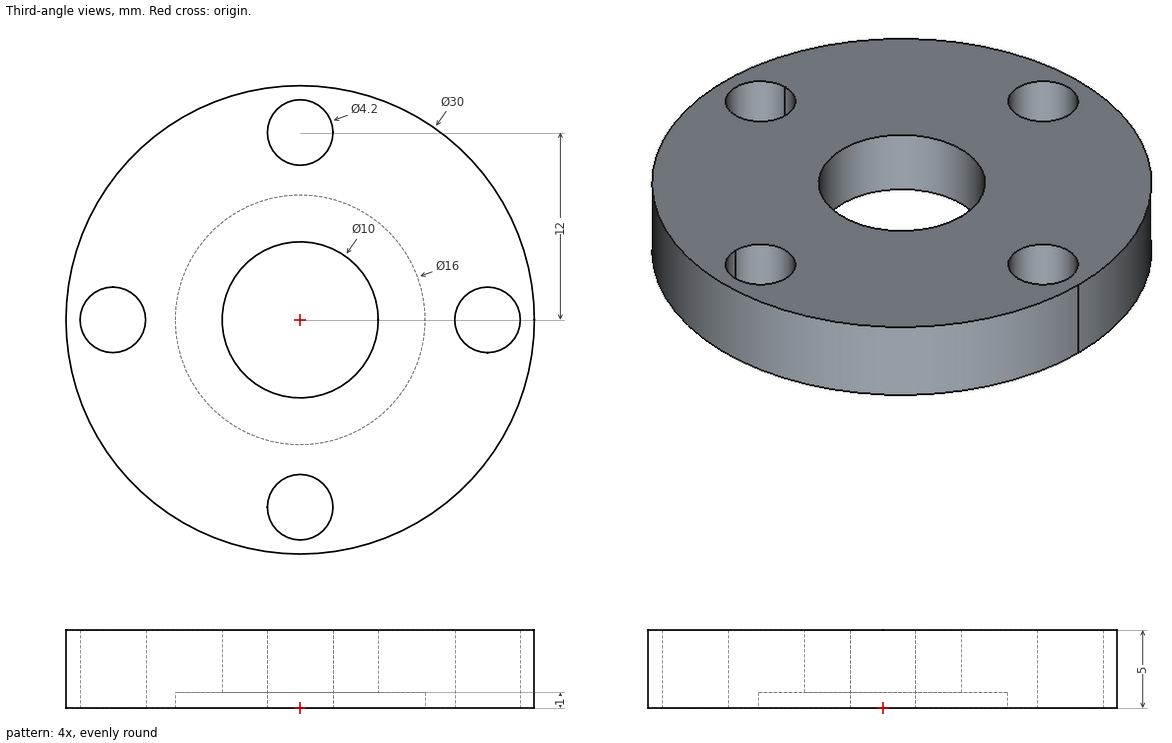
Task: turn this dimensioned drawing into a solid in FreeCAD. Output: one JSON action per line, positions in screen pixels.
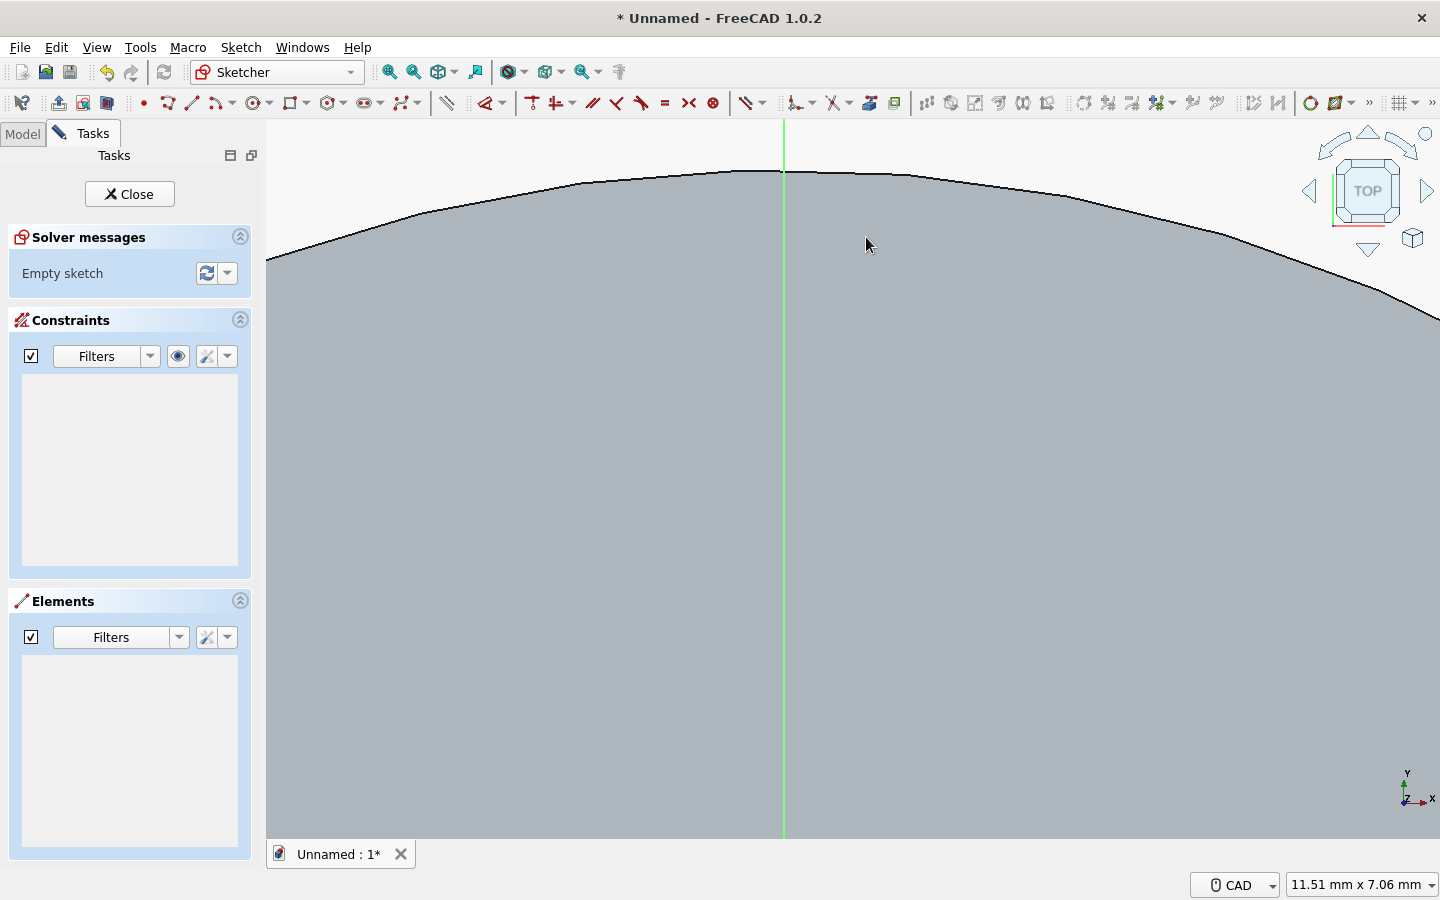
{"action": "left_click", "coordinate": [254, 104]}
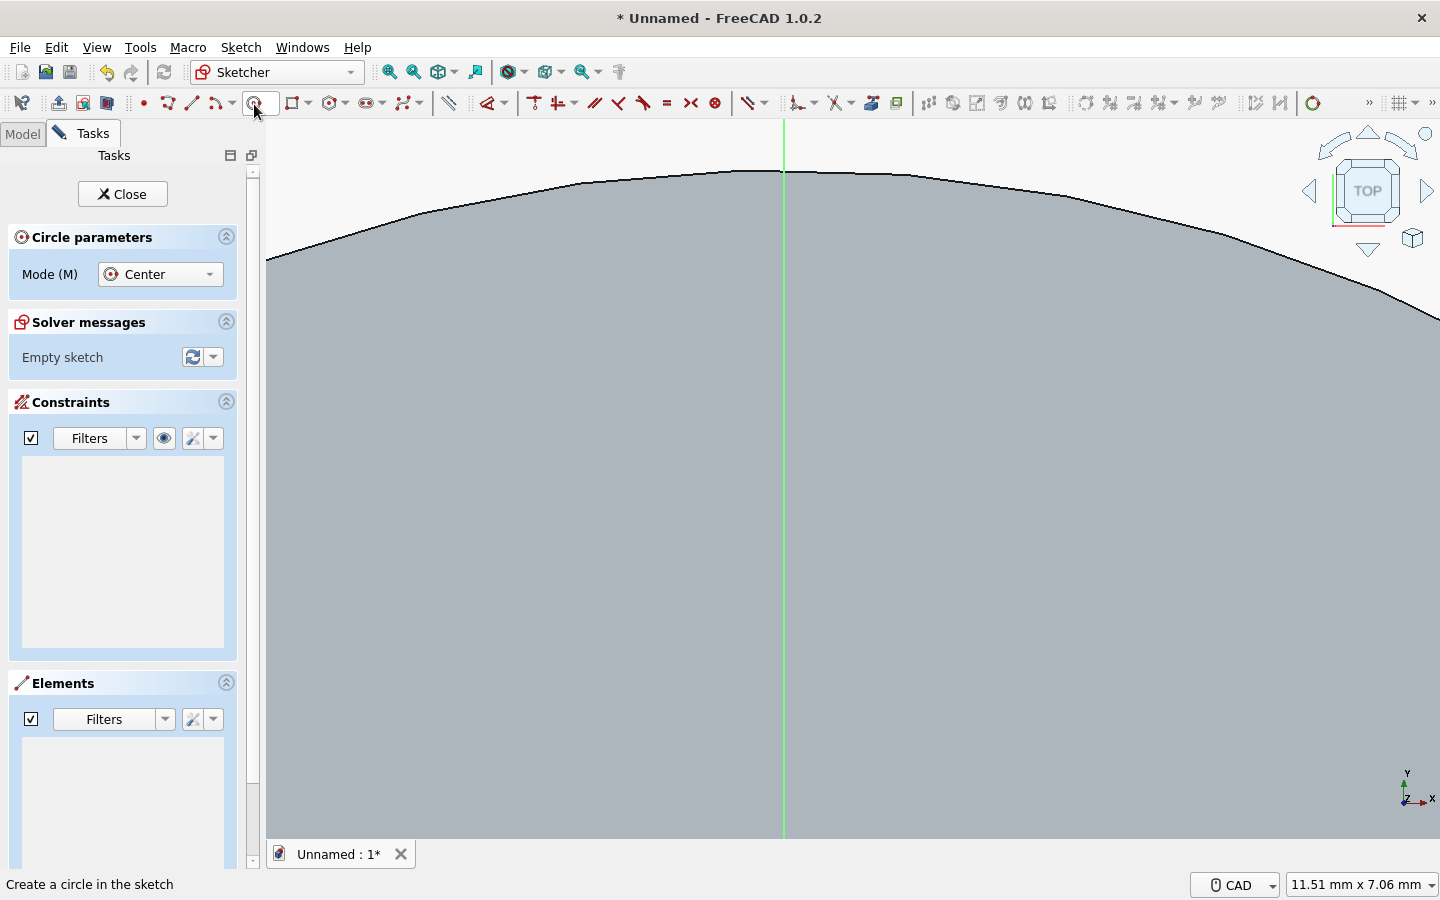
{"action": "left_click", "coordinate": [784, 476]}
{"action": "mouse_move", "coordinate": [935, 325]}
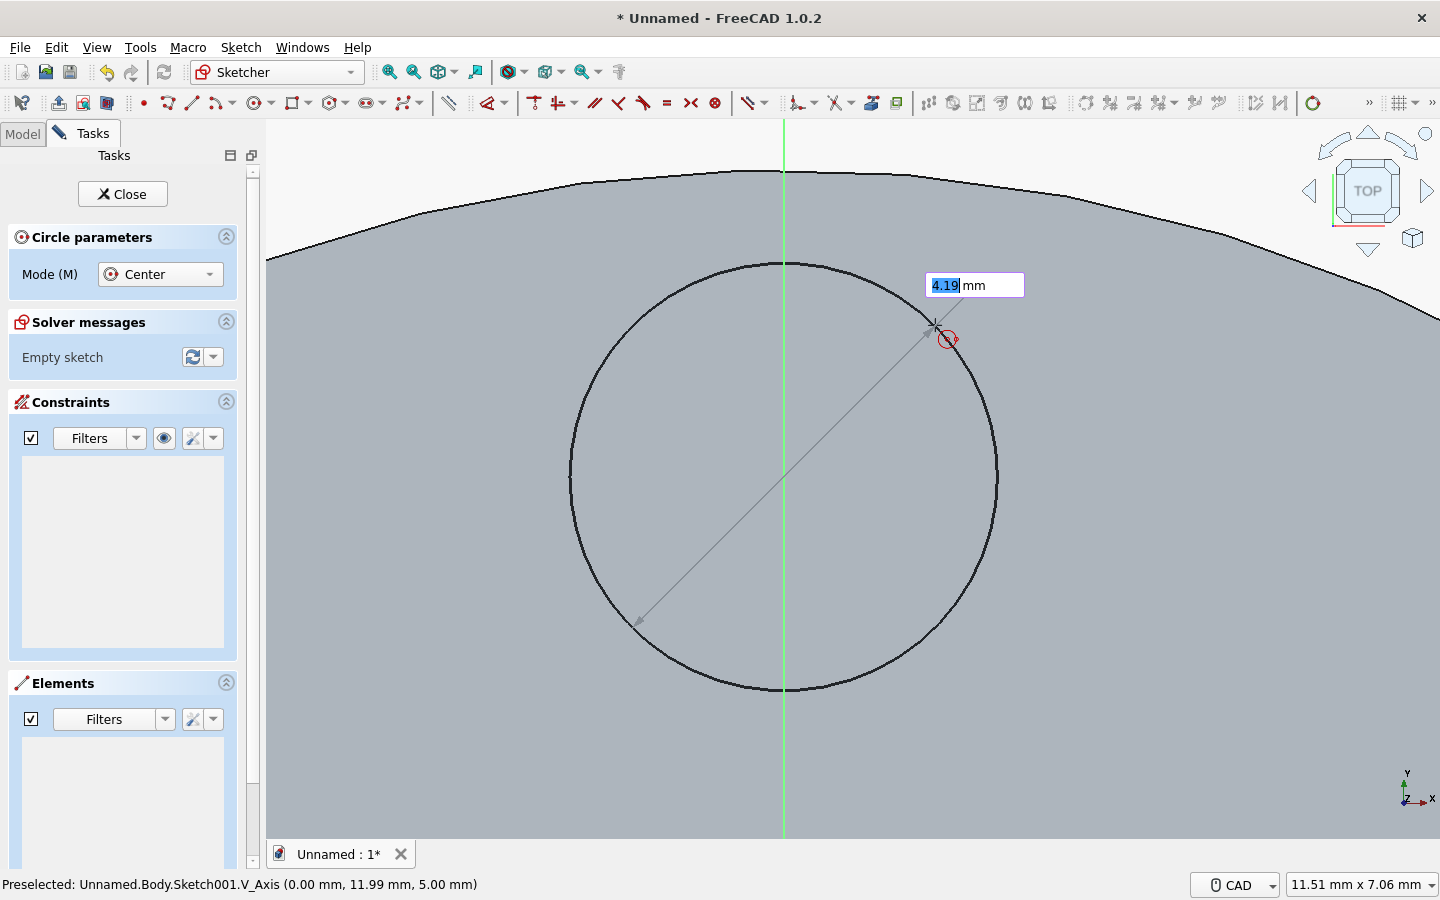
{"action": "type", "text": "4.2"}
{"action": "key", "text": "Return"}
{"action": "key", "text": "Escape"}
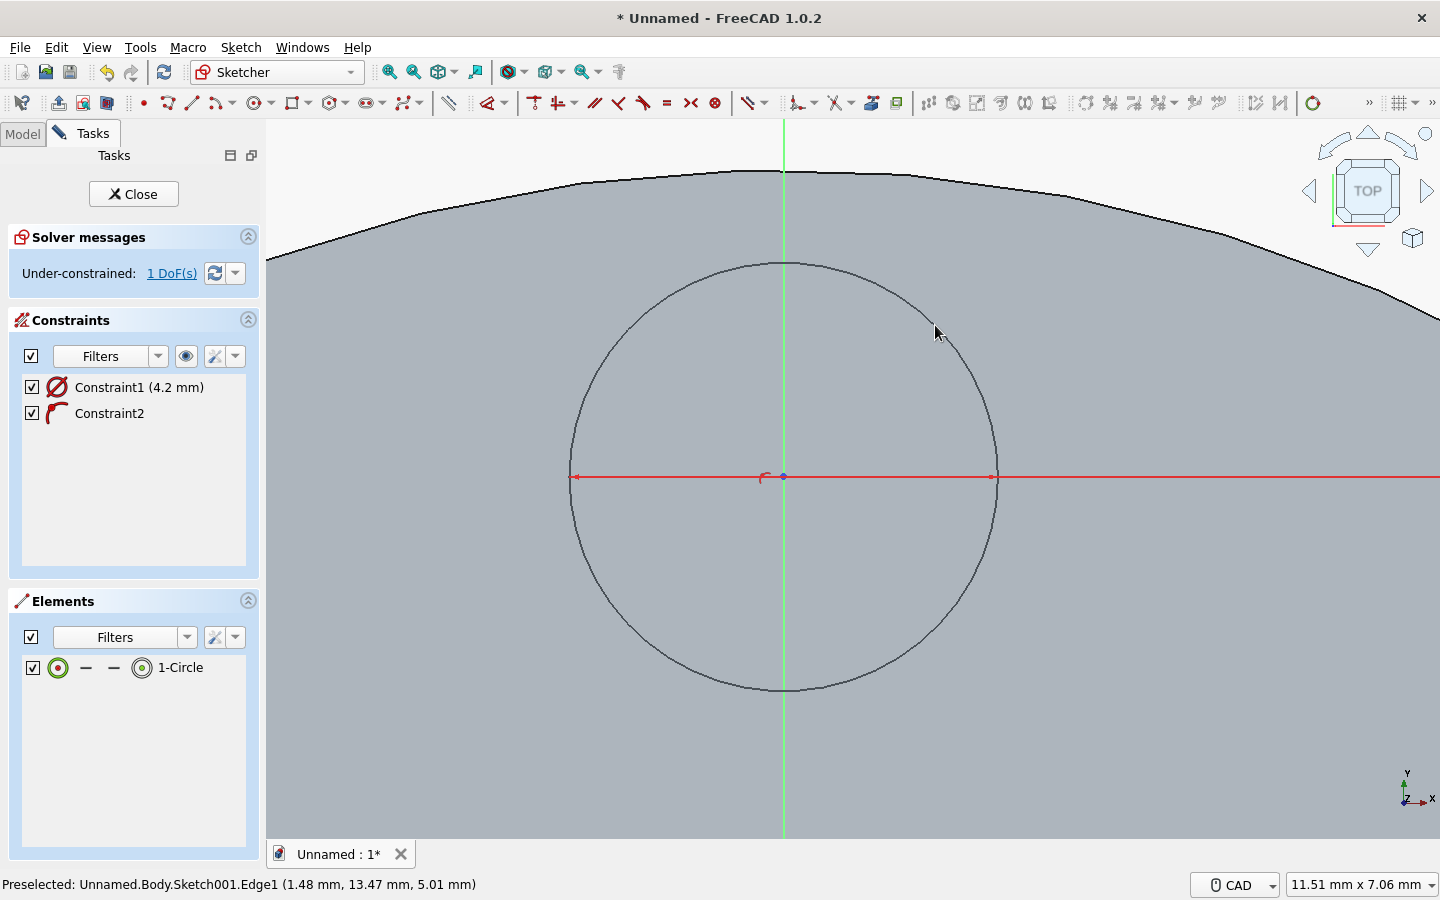
{"action": "left_click", "coordinate": [784, 477]}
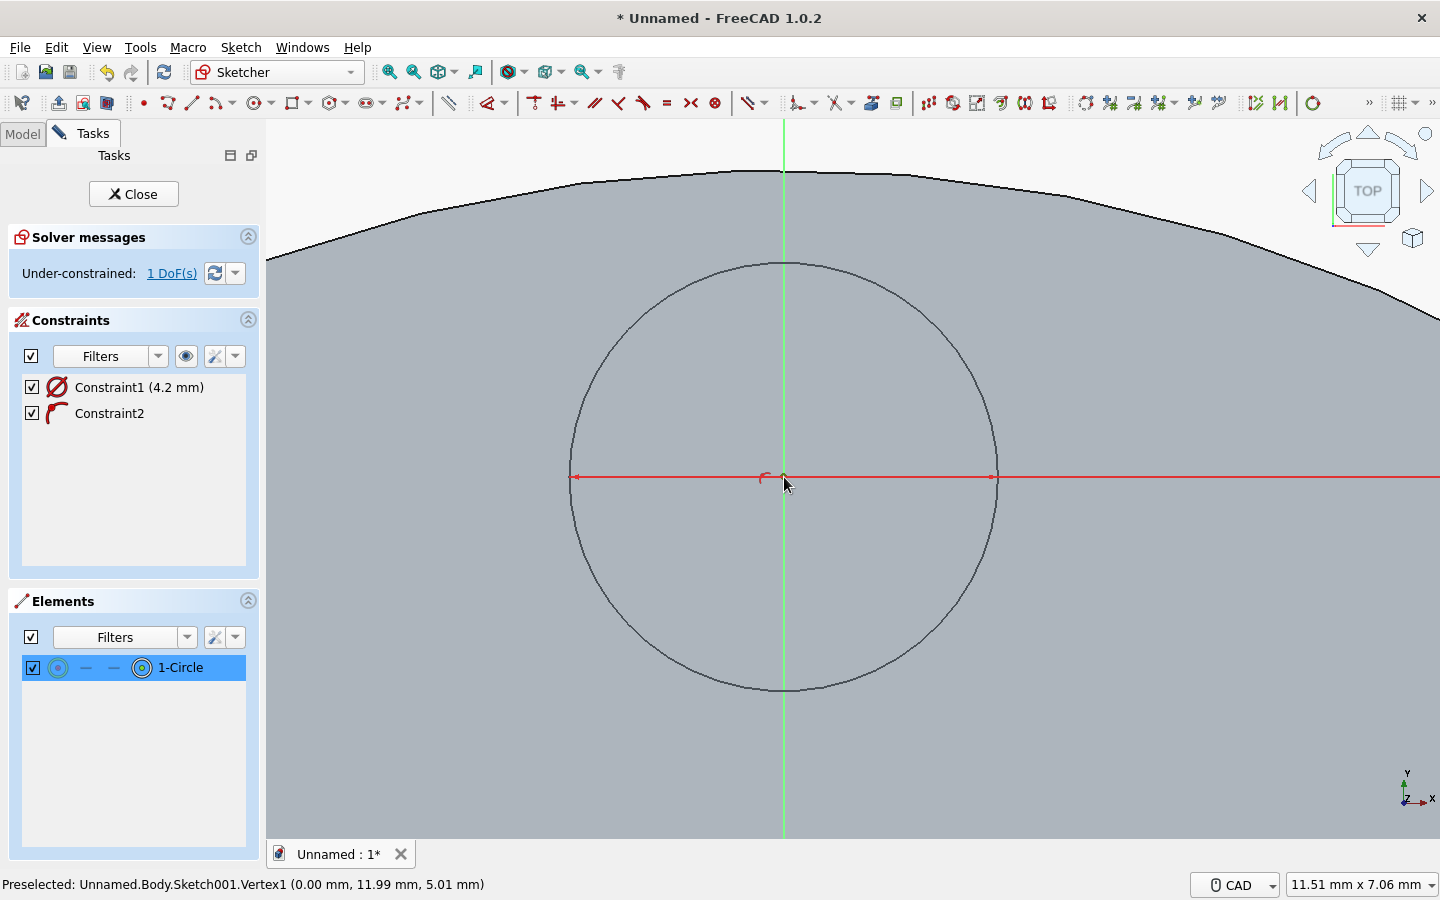
{"action": "key", "text": "i"}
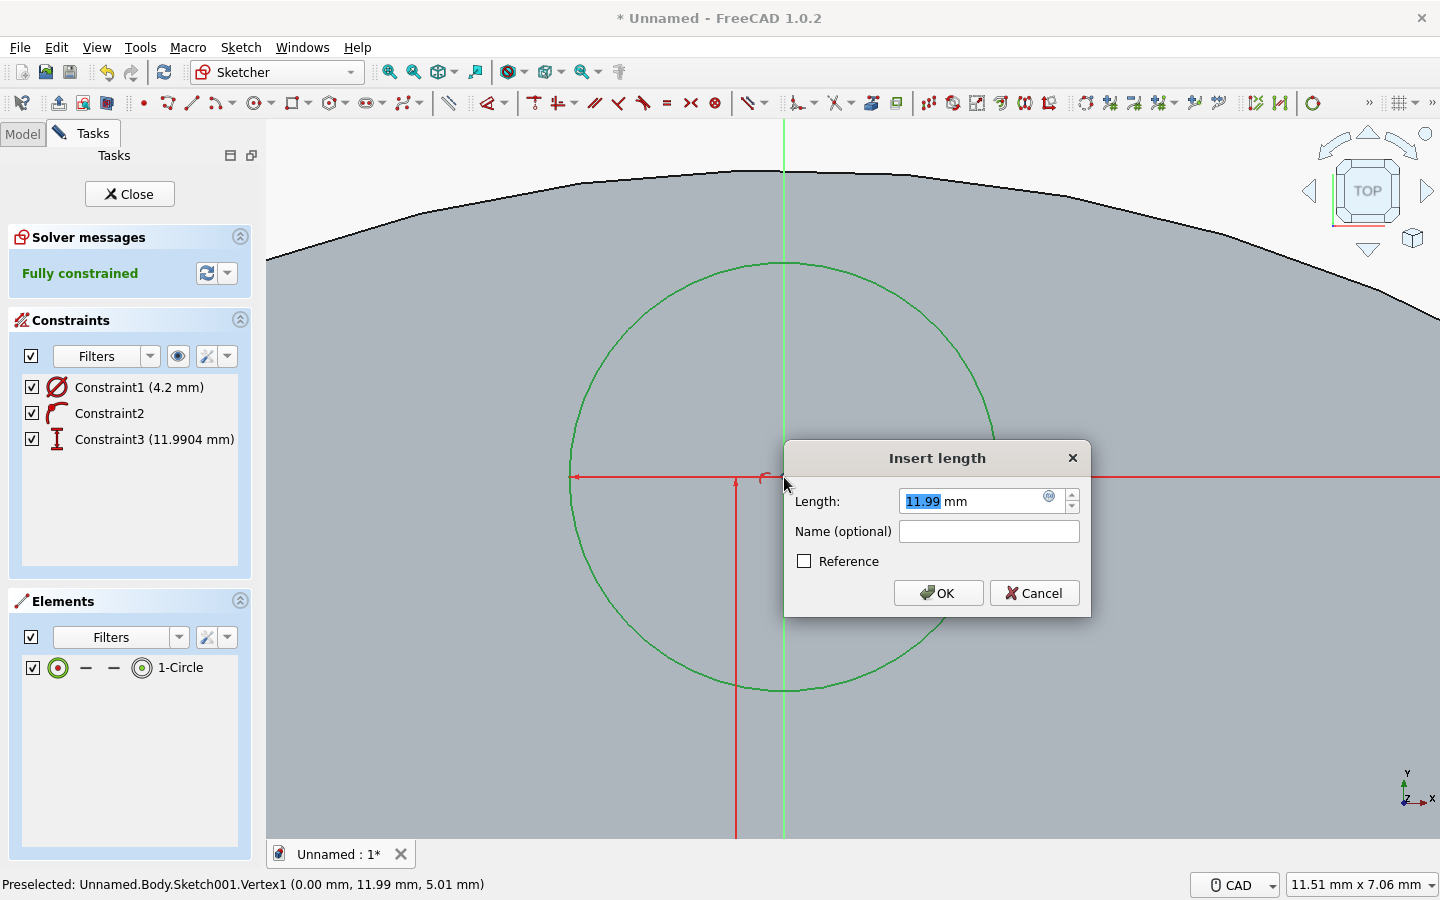
{"action": "type", "text": "12"}
{"action": "key", "text": "Return"}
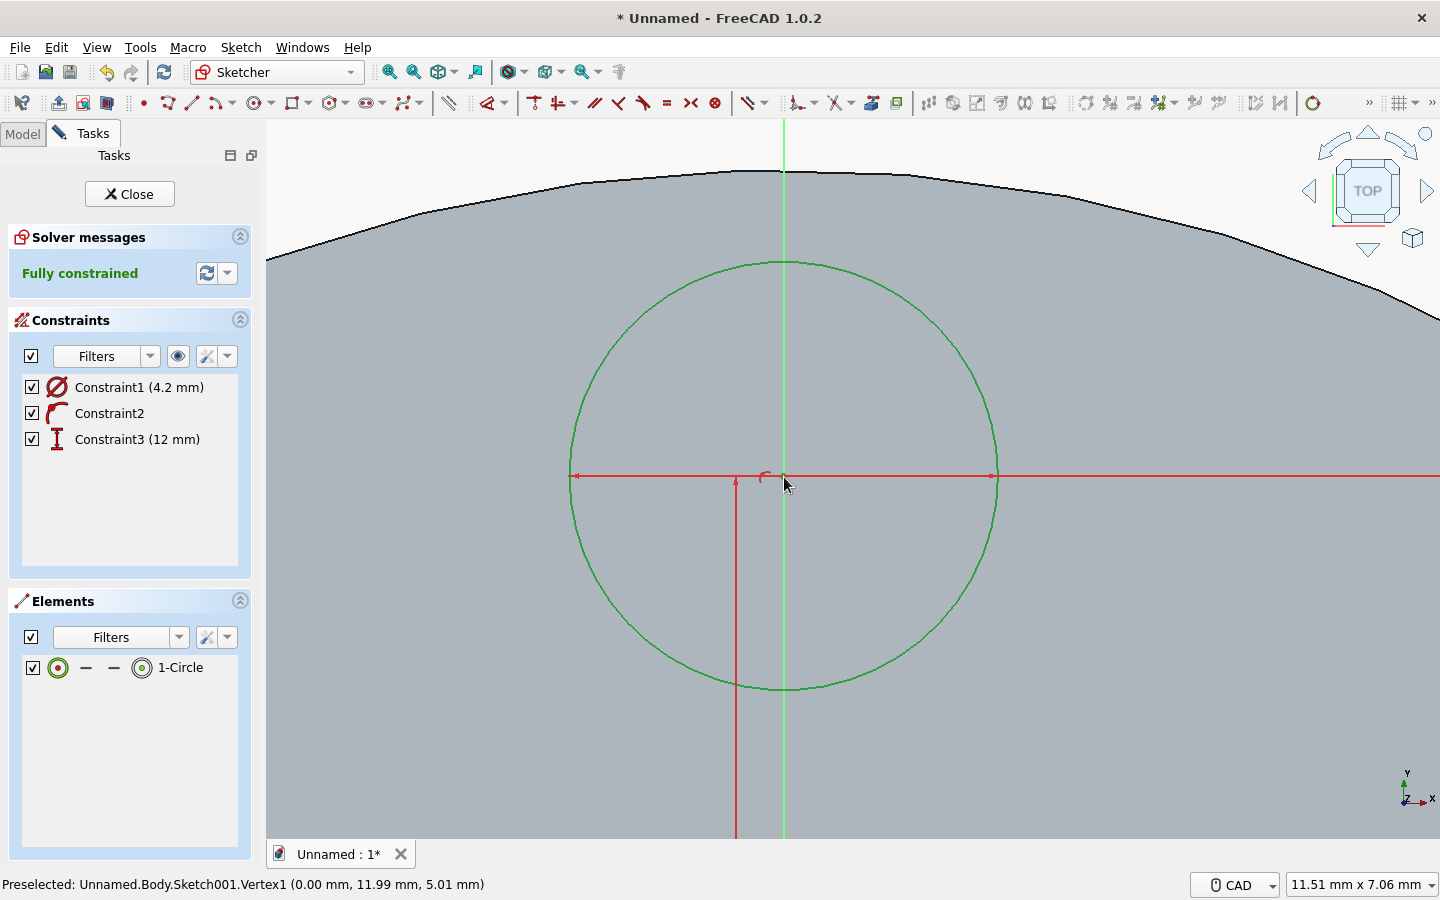
{"action": "left_click", "coordinate": [130, 194]}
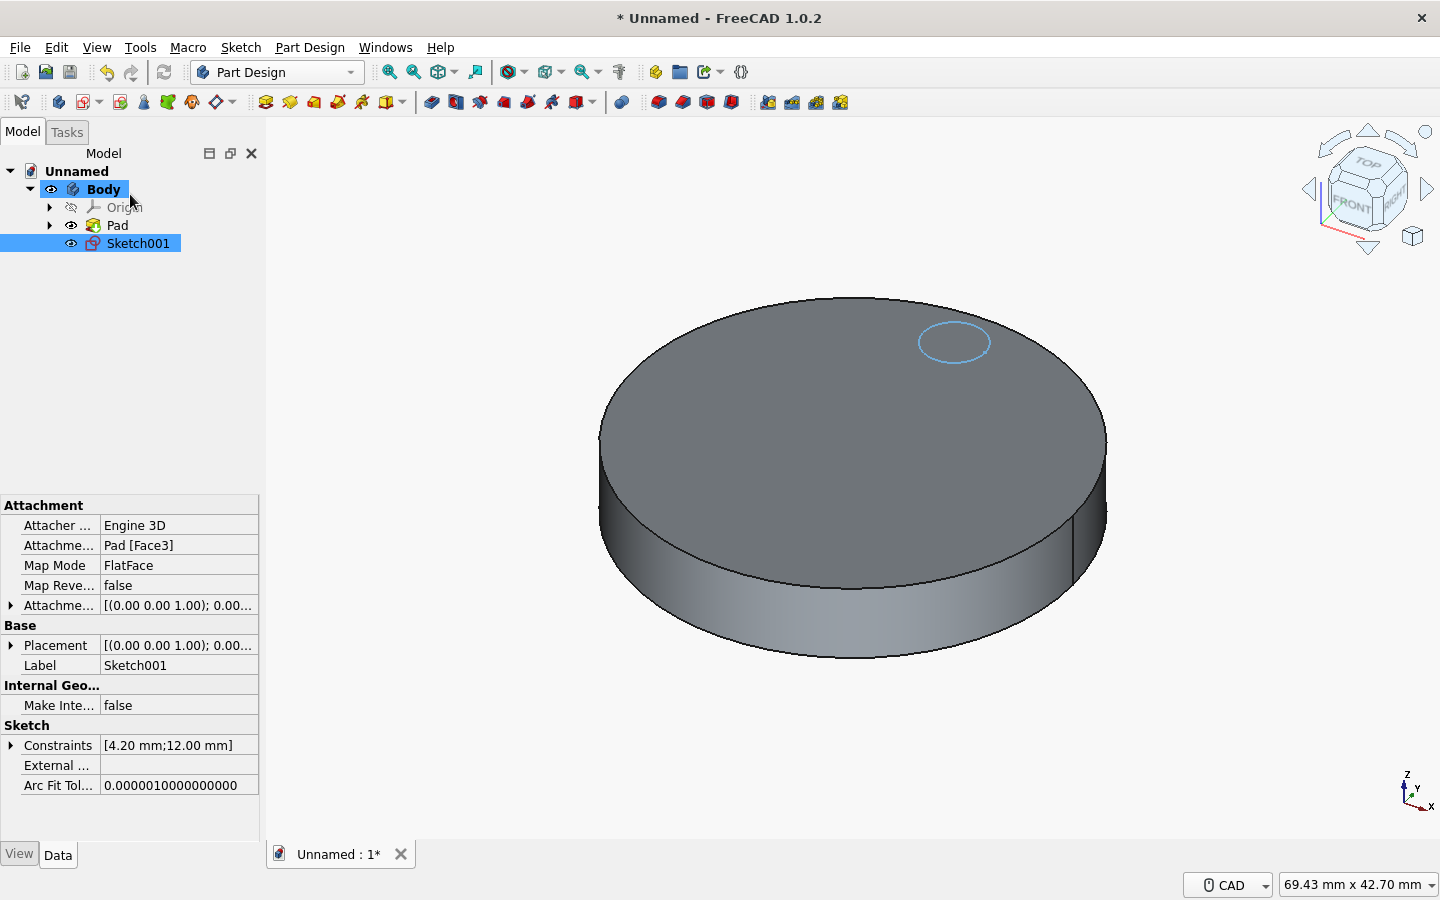
{"action": "left_click", "coordinate": [432, 102]}